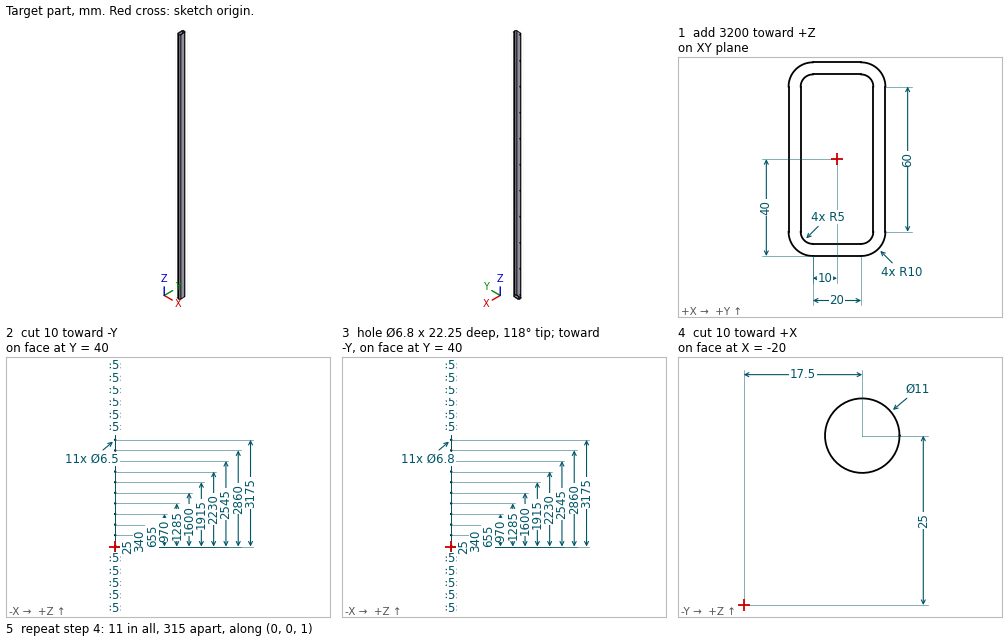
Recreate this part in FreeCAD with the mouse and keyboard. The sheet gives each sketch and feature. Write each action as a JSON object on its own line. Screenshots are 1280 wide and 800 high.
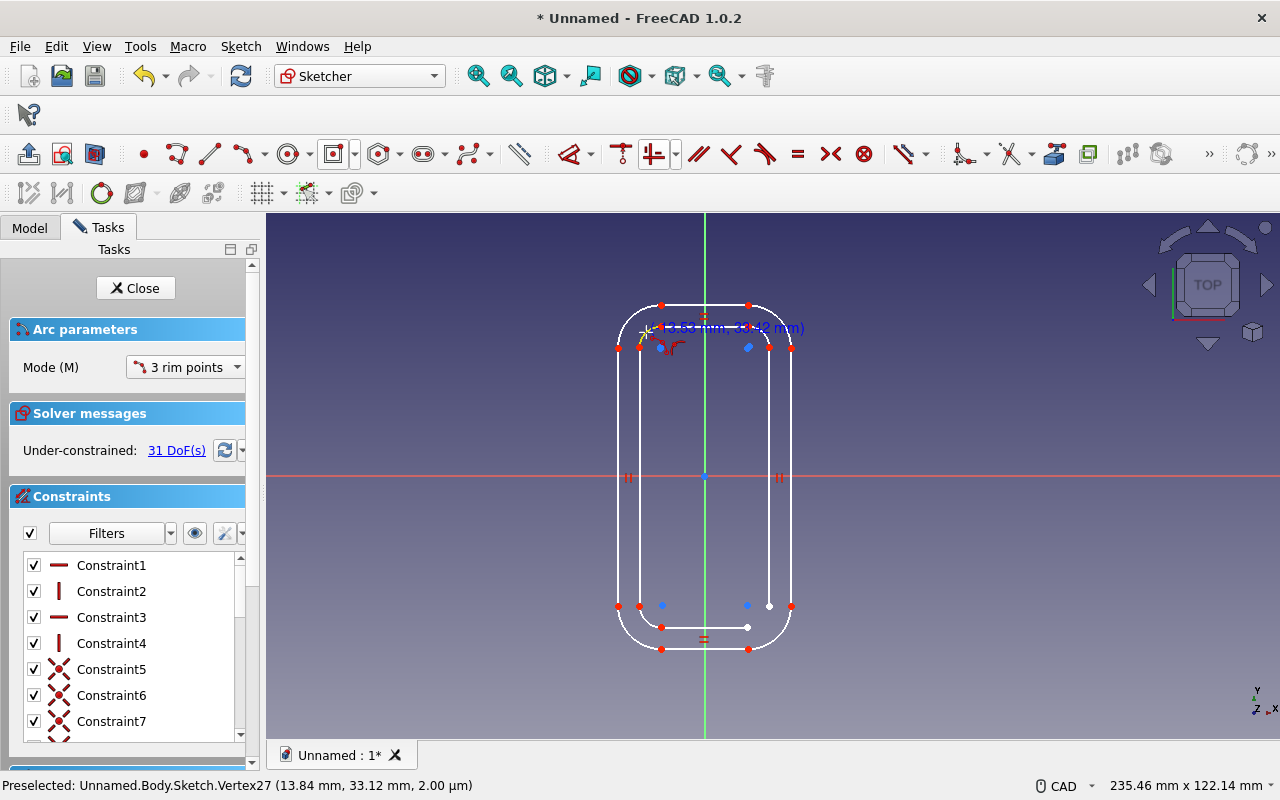
{"action": "left_click", "coordinate": [769, 607]}
{"action": "left_click", "coordinate": [748, 628]}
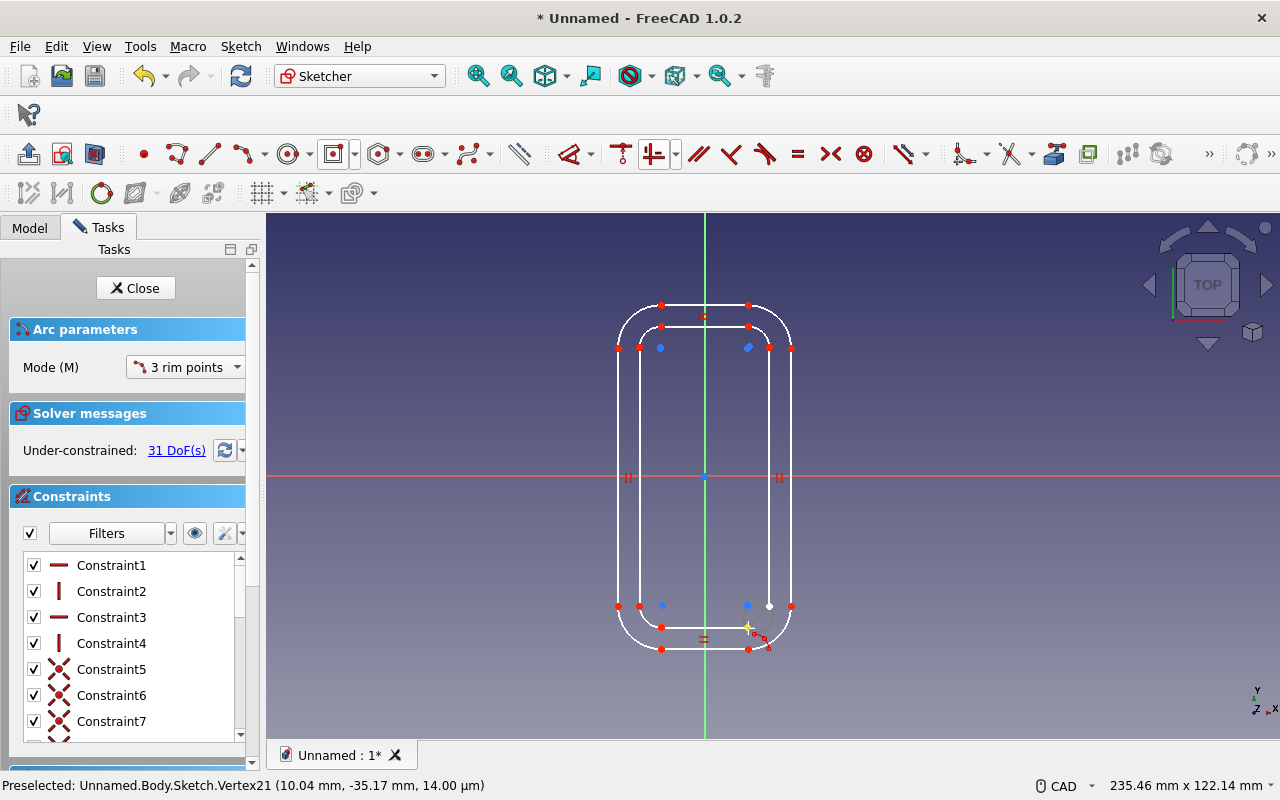
{"action": "scroll", "coordinate": [763, 621], "scroll_direction": "up", "scroll_amount": 5}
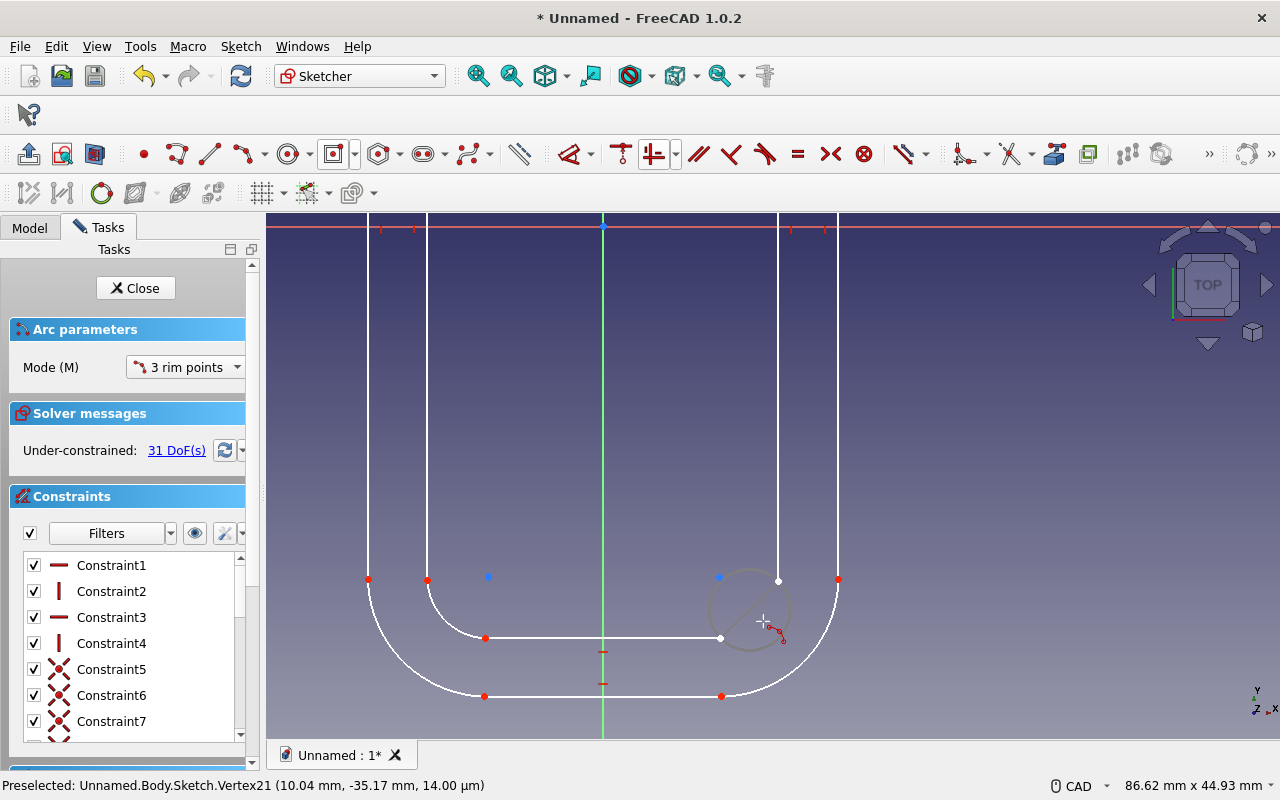
{"action": "left_click", "coordinate": [762, 619]}
{"action": "key", "text": "Escape"}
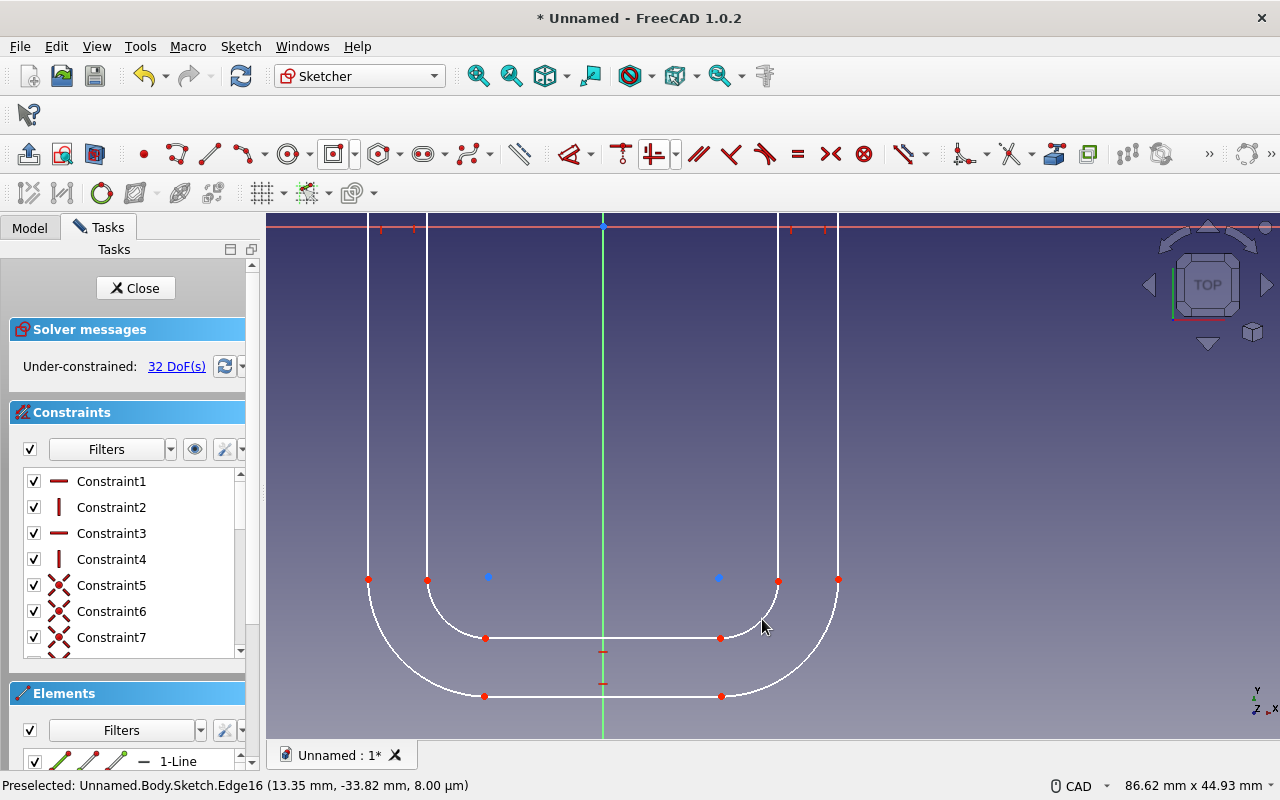
{"action": "left_click", "coordinate": [556, 697]}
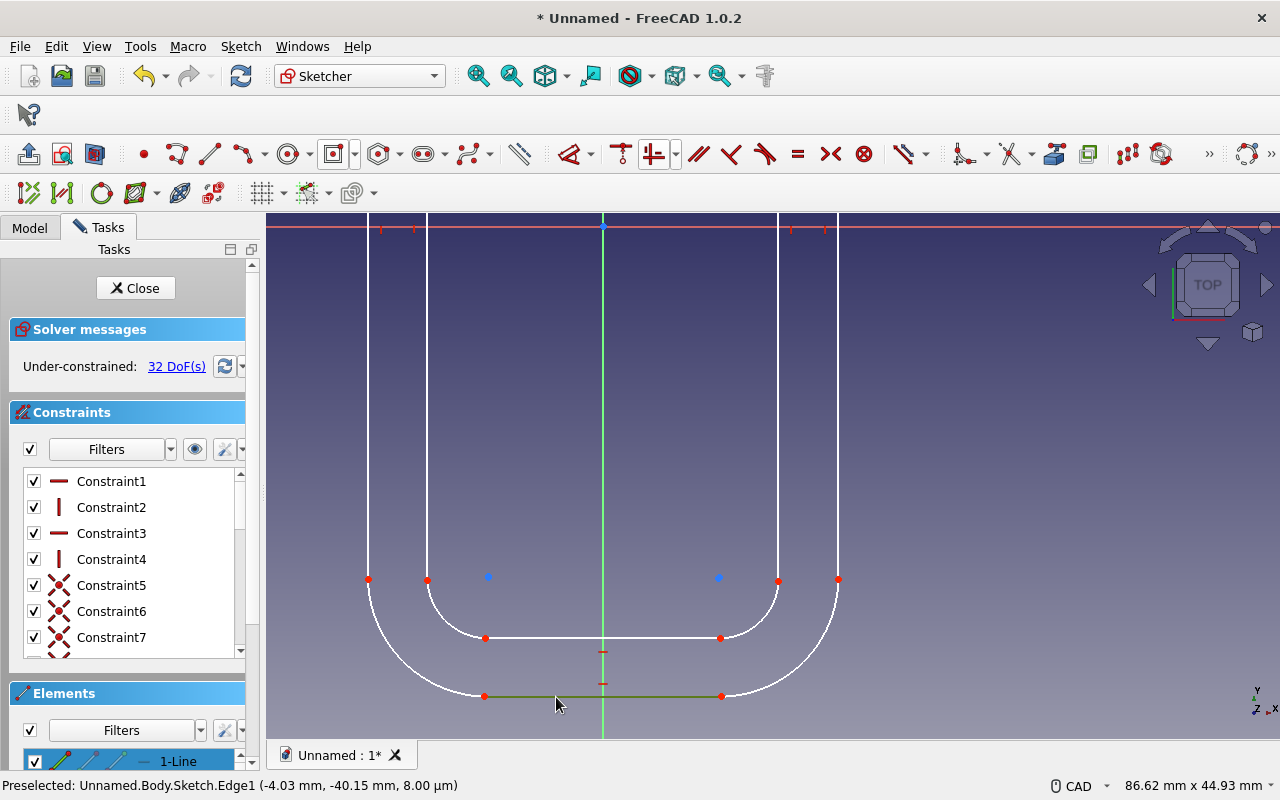
{"action": "left_click", "coordinate": [774, 683]}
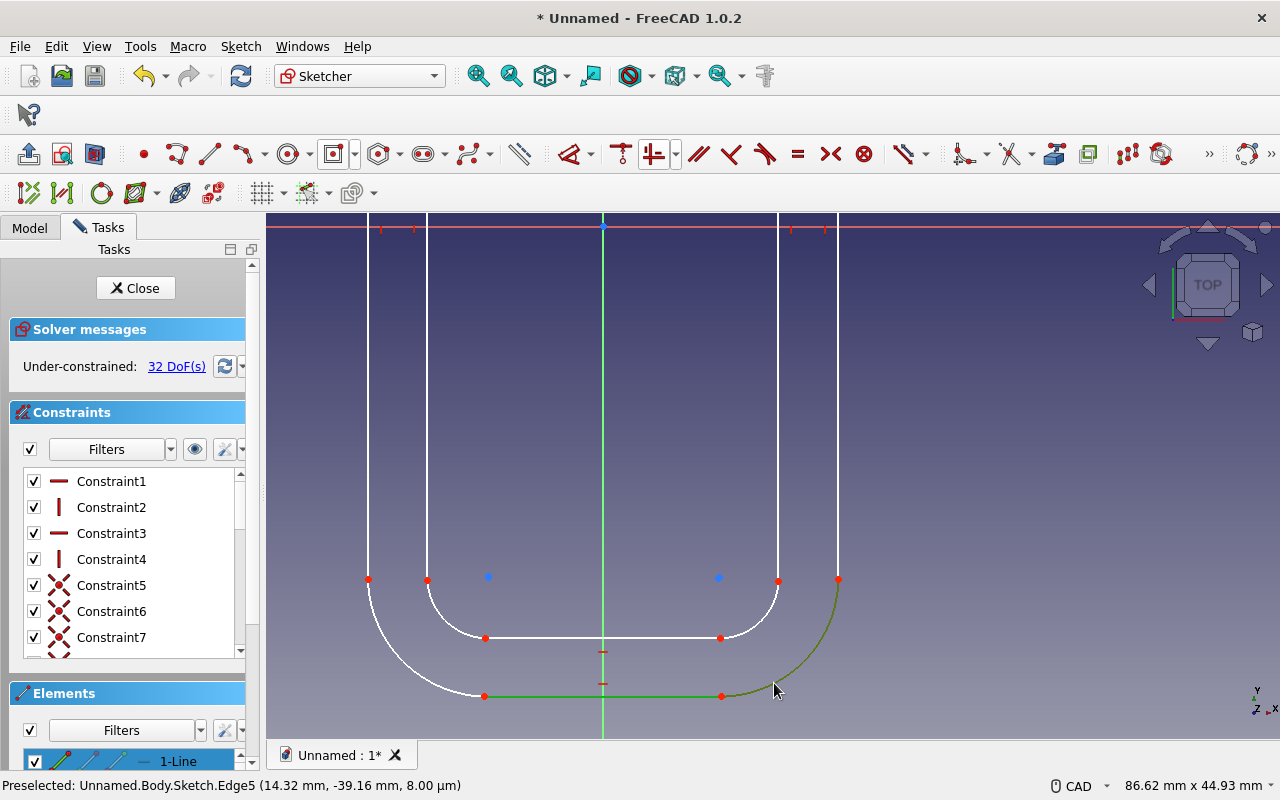
{"action": "left_click", "coordinate": [765, 154]}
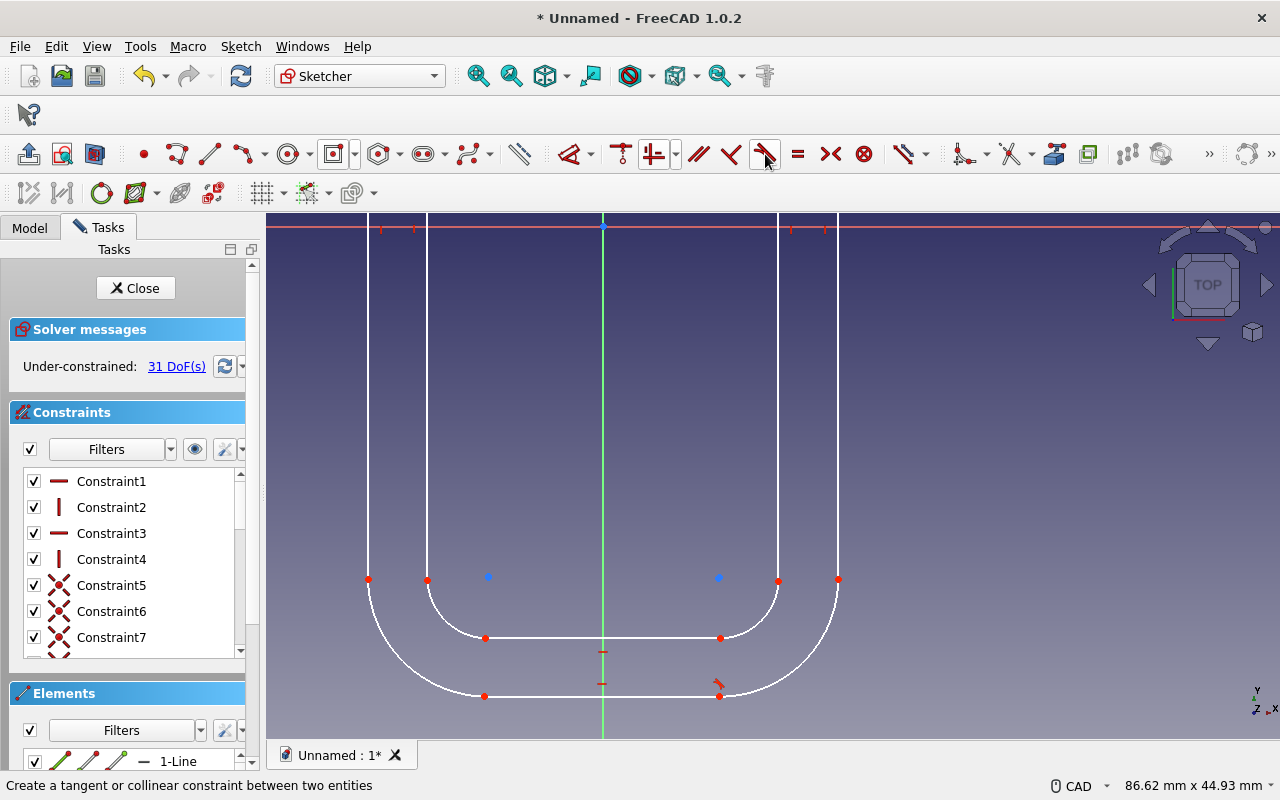
{"action": "left_click", "coordinate": [555, 697]}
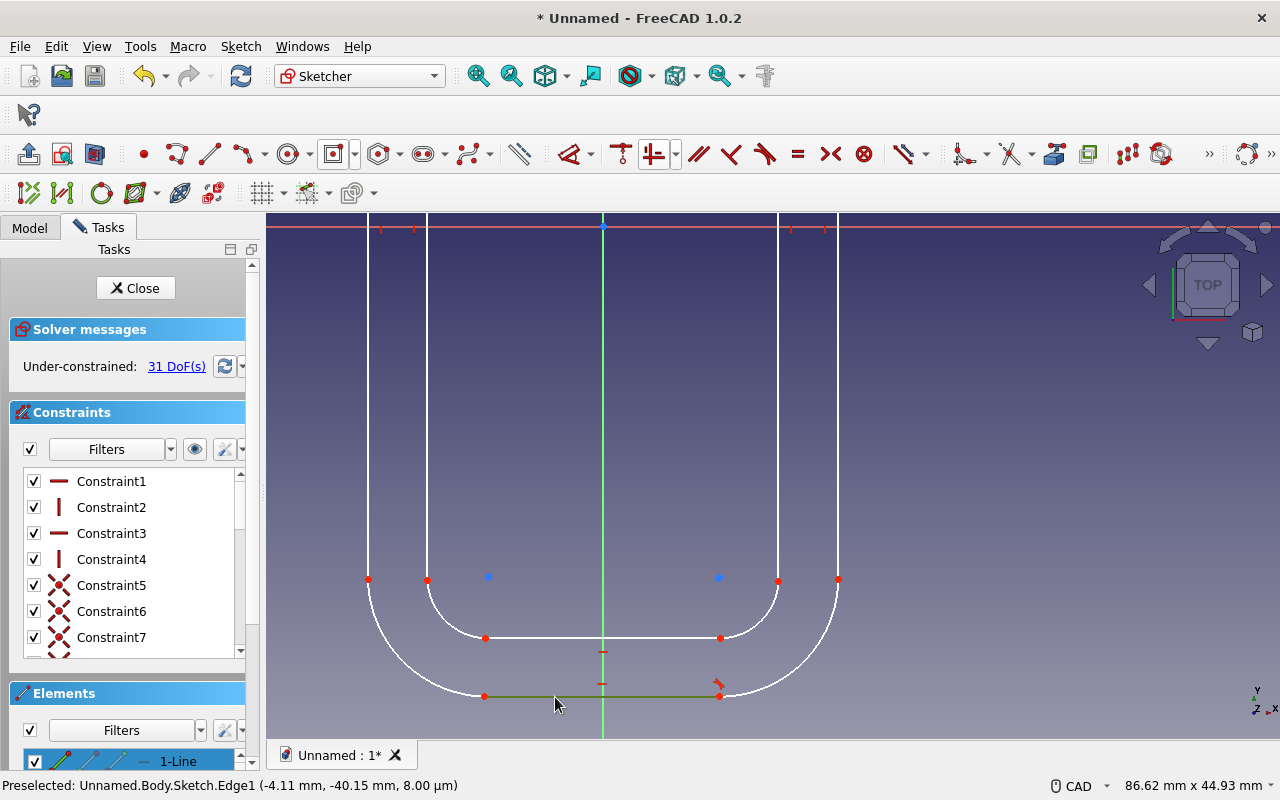
{"action": "left_click", "coordinate": [382, 632]}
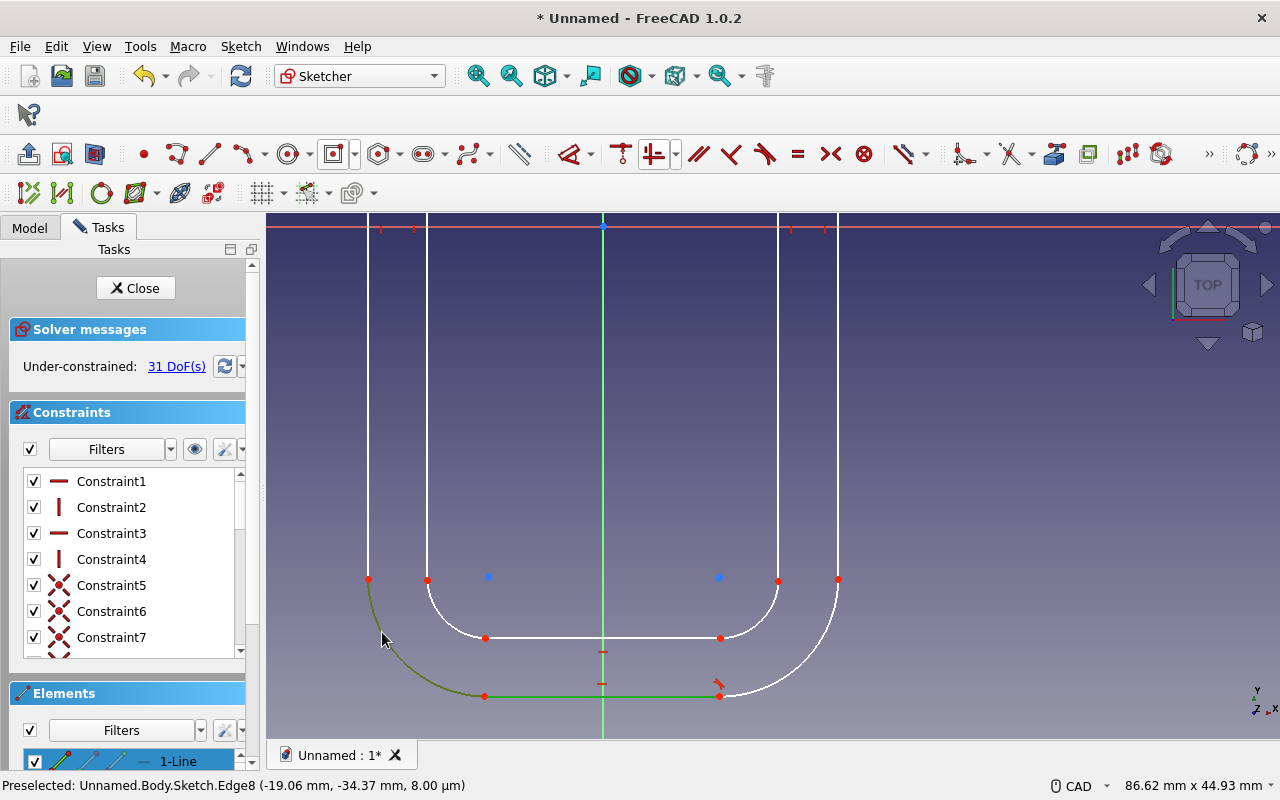
{"action": "left_click", "coordinate": [765, 154]}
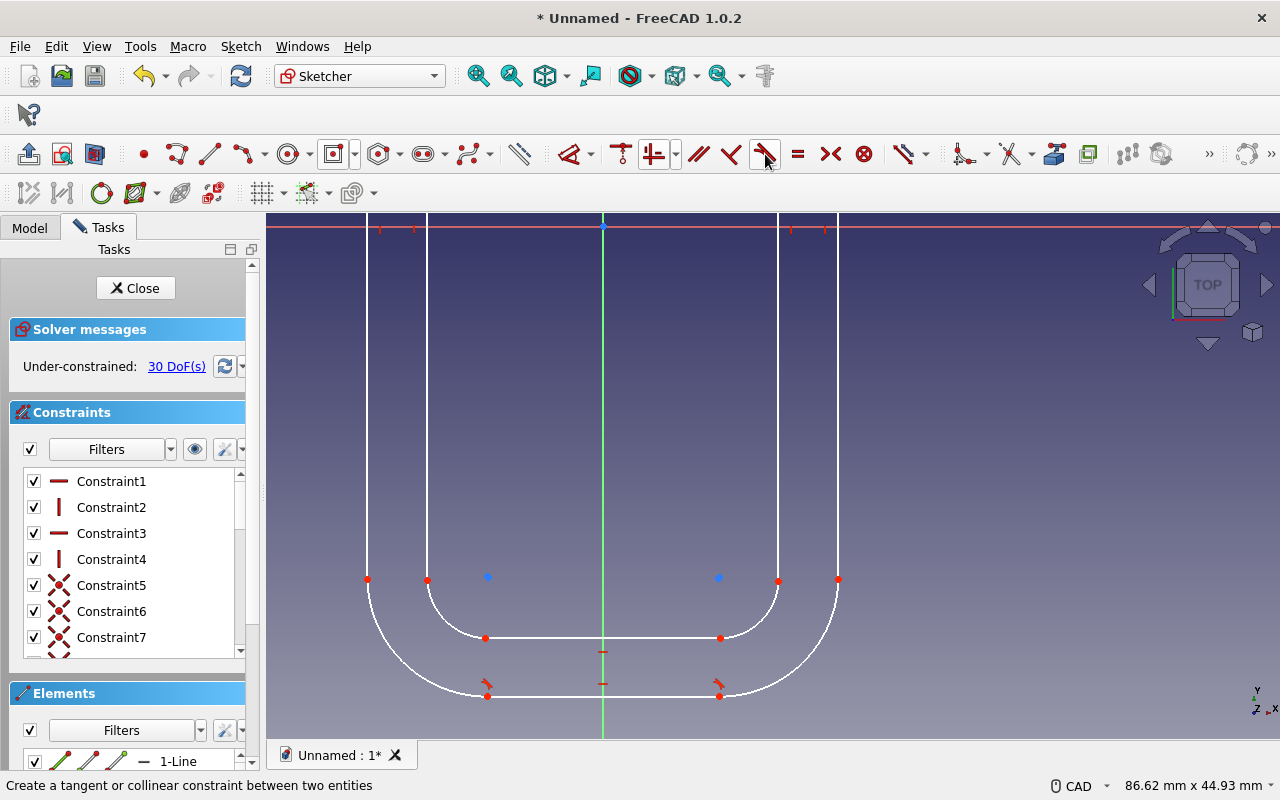
{"action": "left_click", "coordinate": [838, 369]}